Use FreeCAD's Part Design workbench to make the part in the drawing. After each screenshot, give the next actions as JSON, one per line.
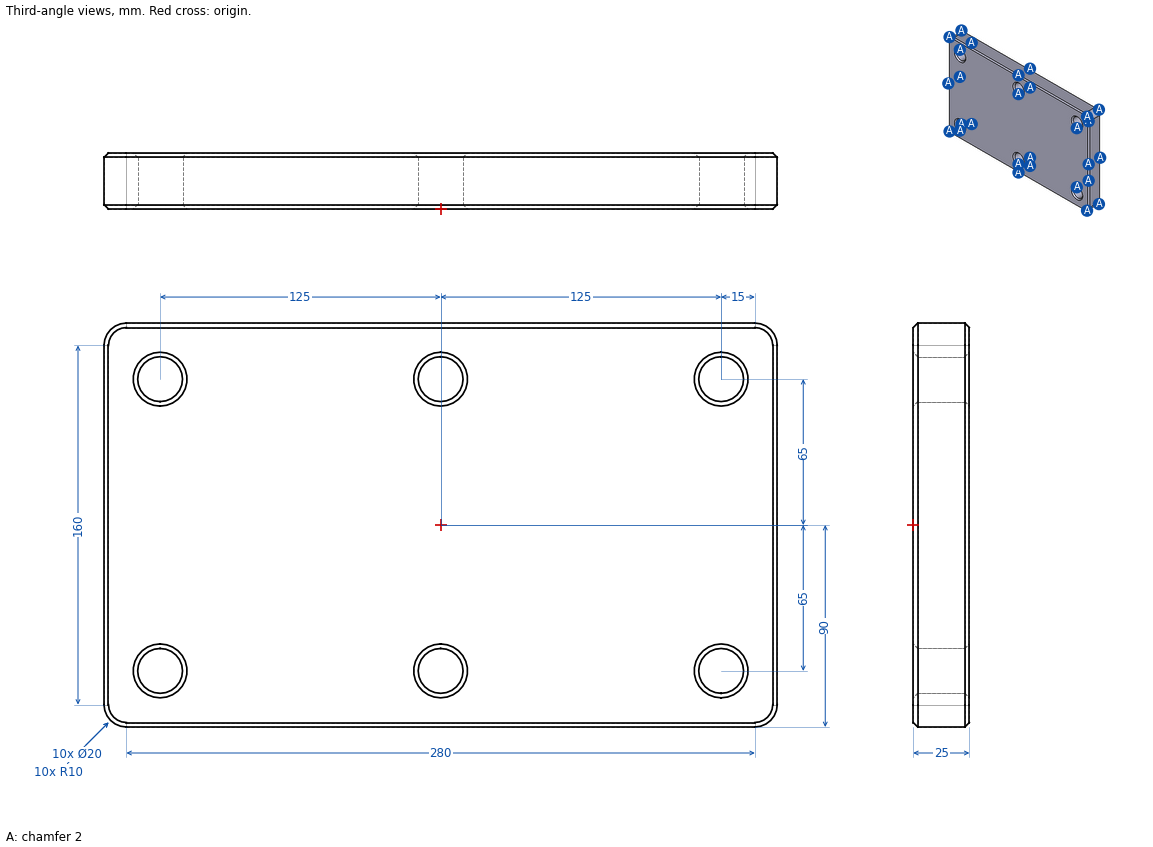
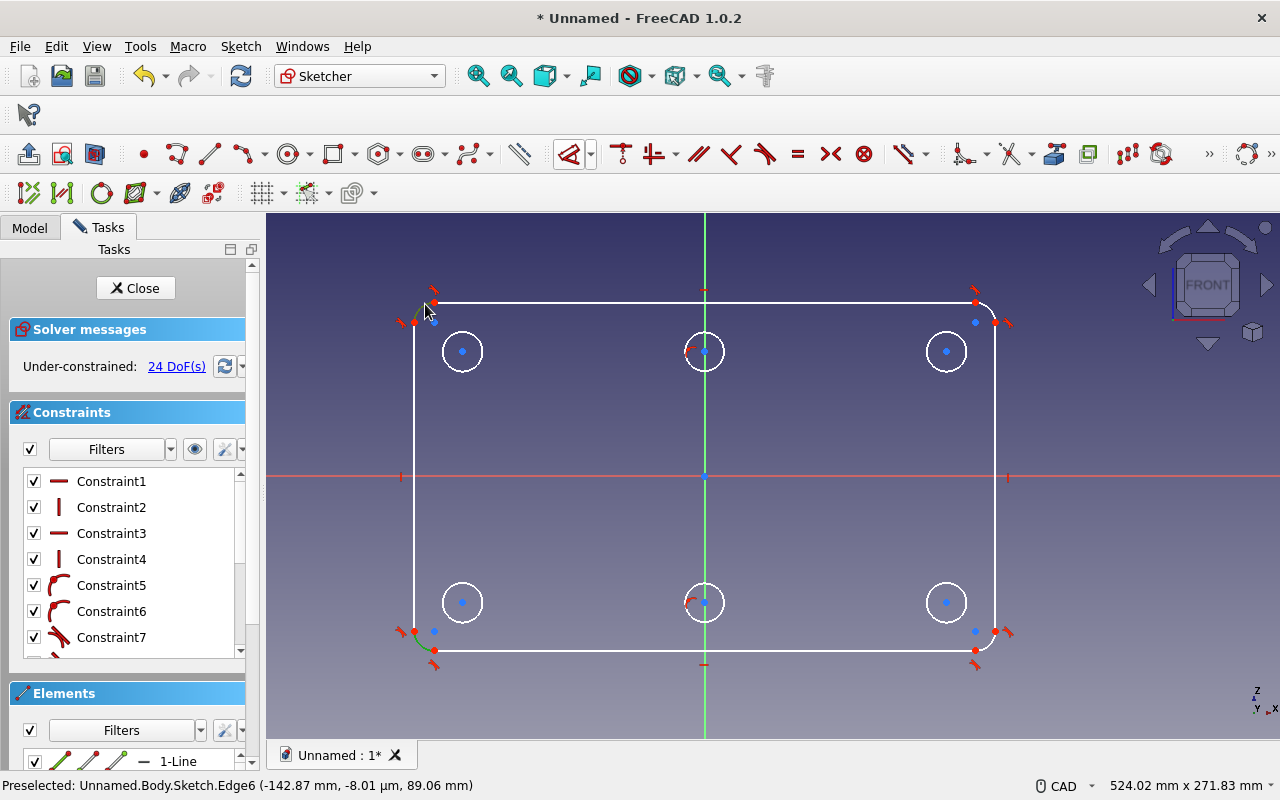
{"action": "scroll", "coordinate": [993, 314], "scroll_direction": "up", "scroll_amount": 2}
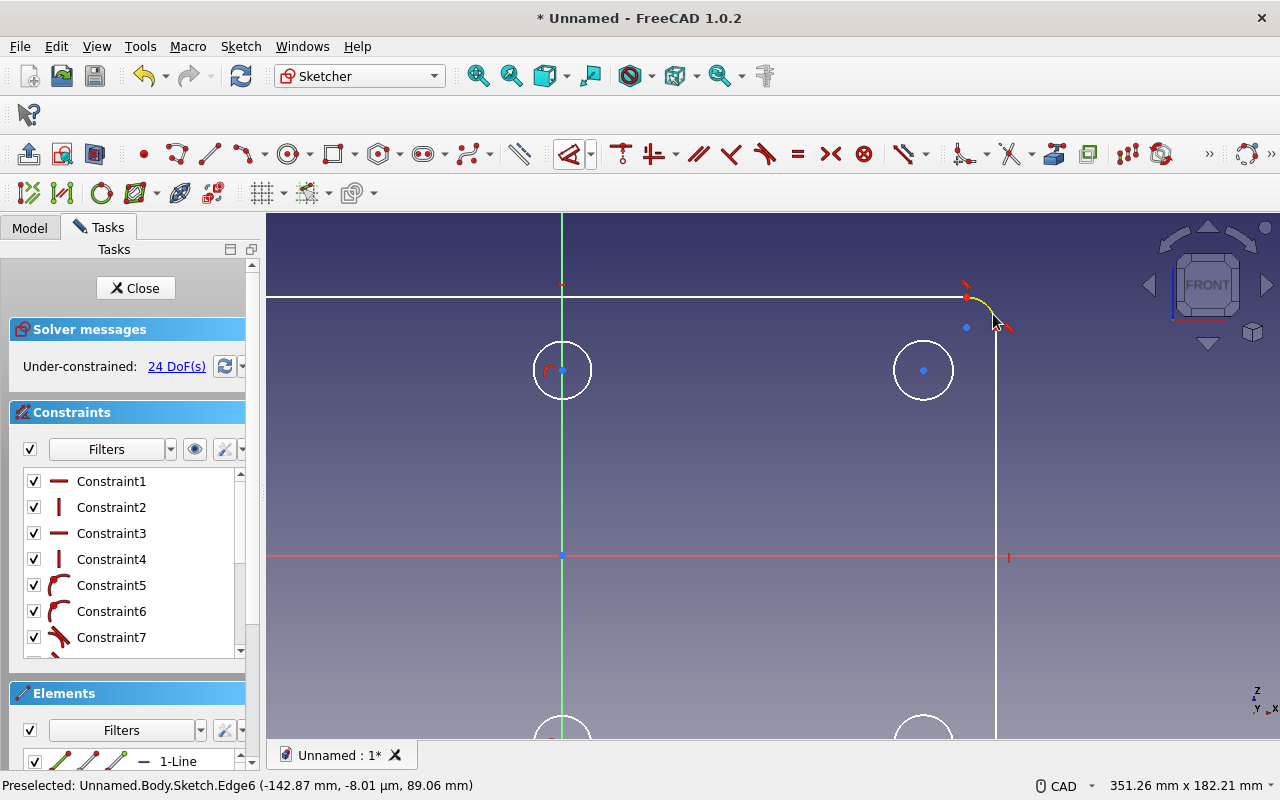
{"action": "left_click", "coordinate": [993, 313]}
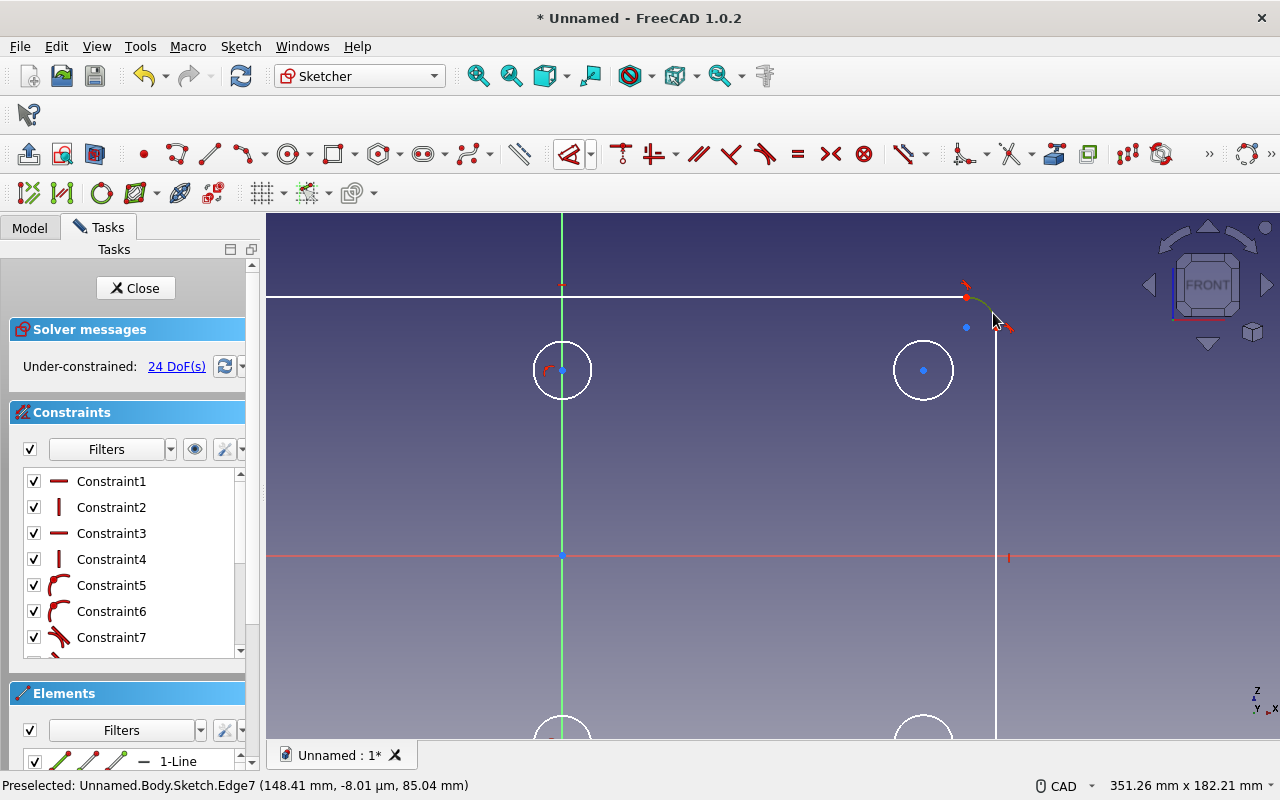
{"action": "scroll", "coordinate": [993, 314], "scroll_direction": "down", "scroll_amount": 2}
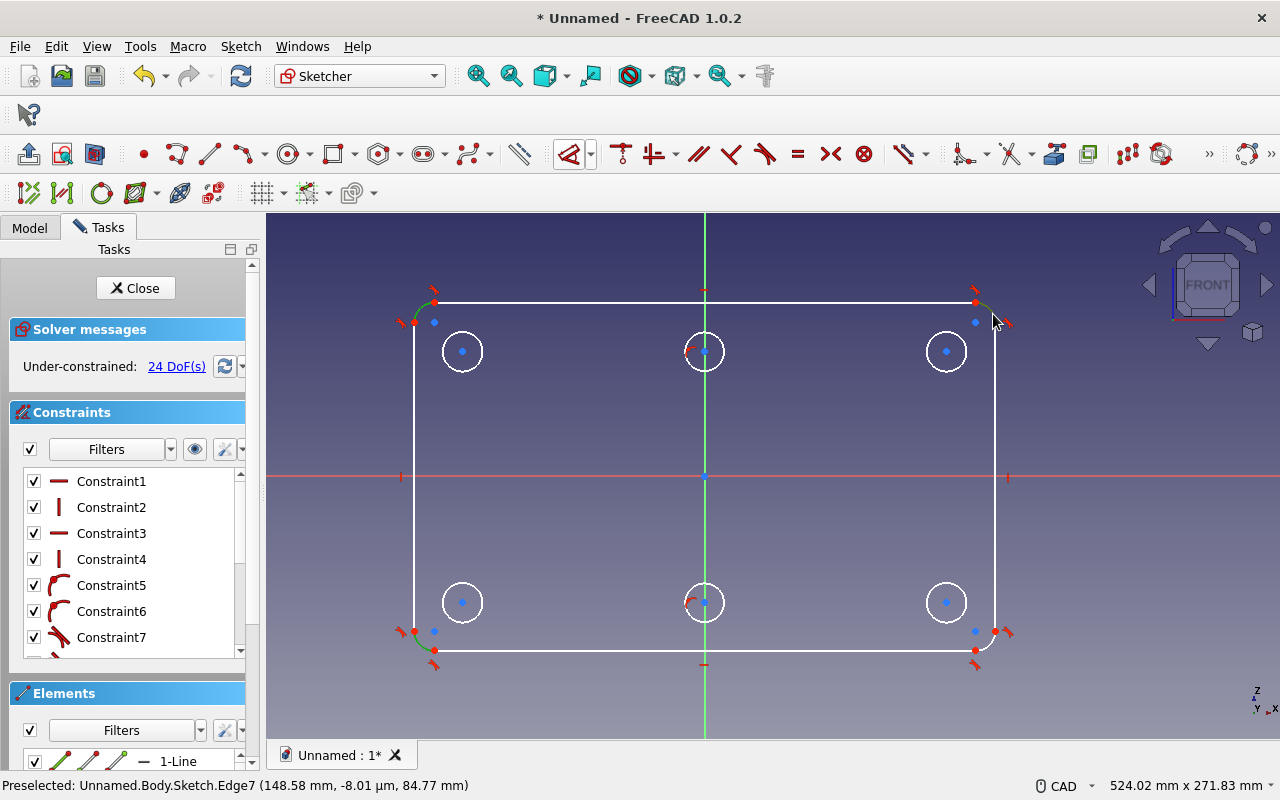
{"action": "scroll", "coordinate": [985, 649], "scroll_direction": "up", "scroll_amount": 3}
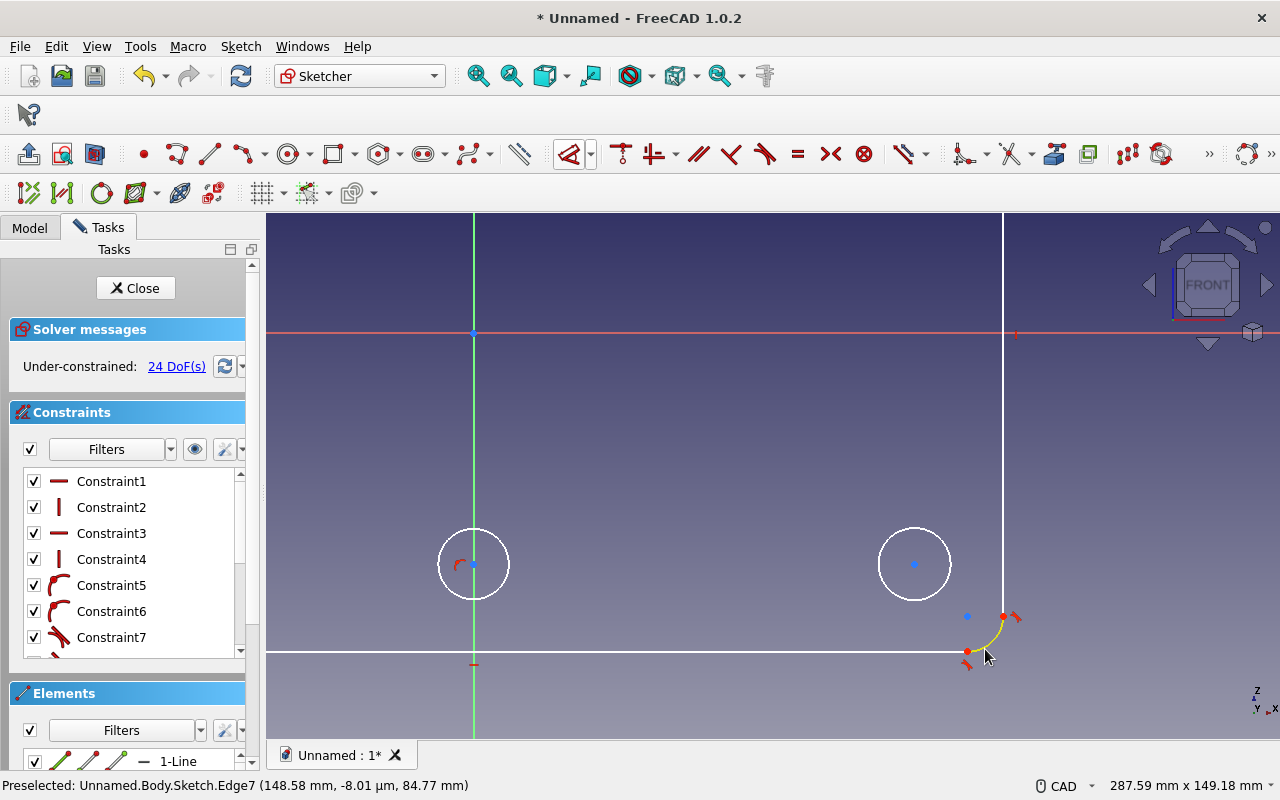
{"action": "left_click", "coordinate": [984, 648]}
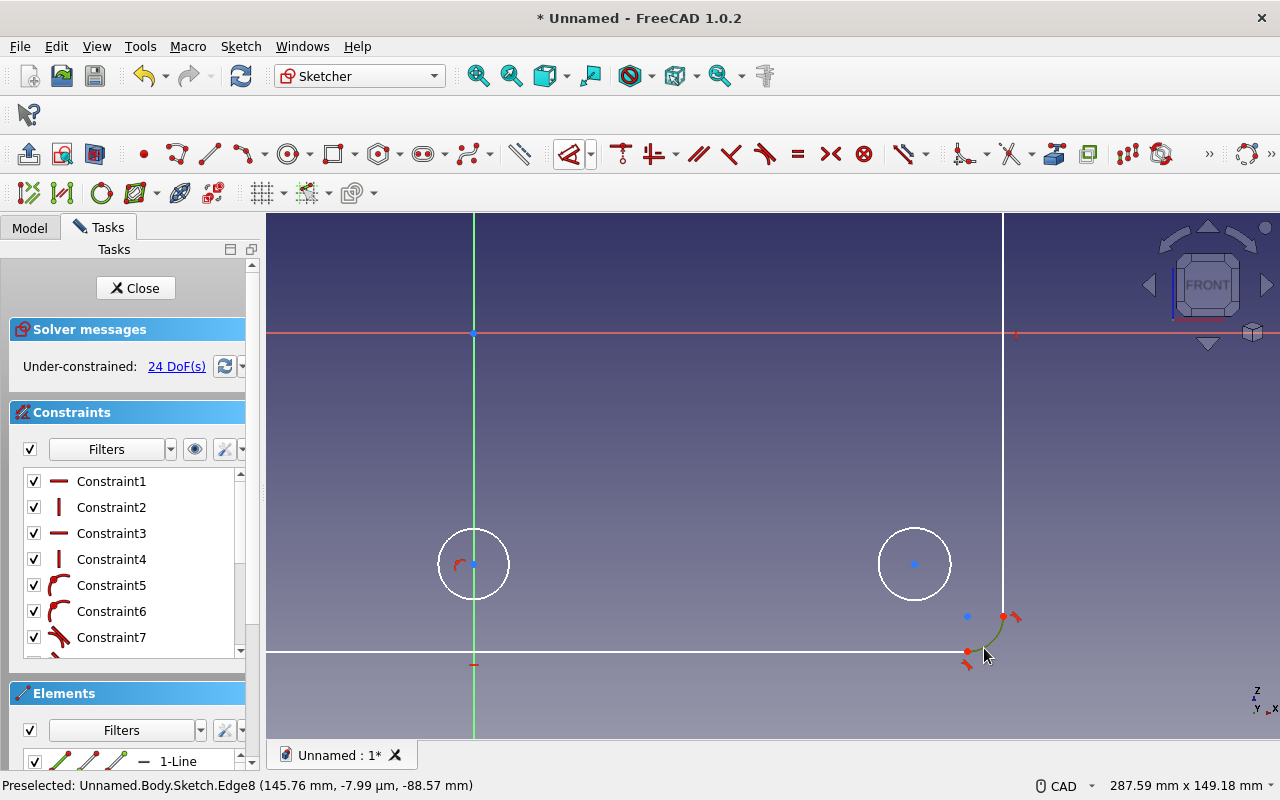
{"action": "left_click", "coordinate": [798, 154]}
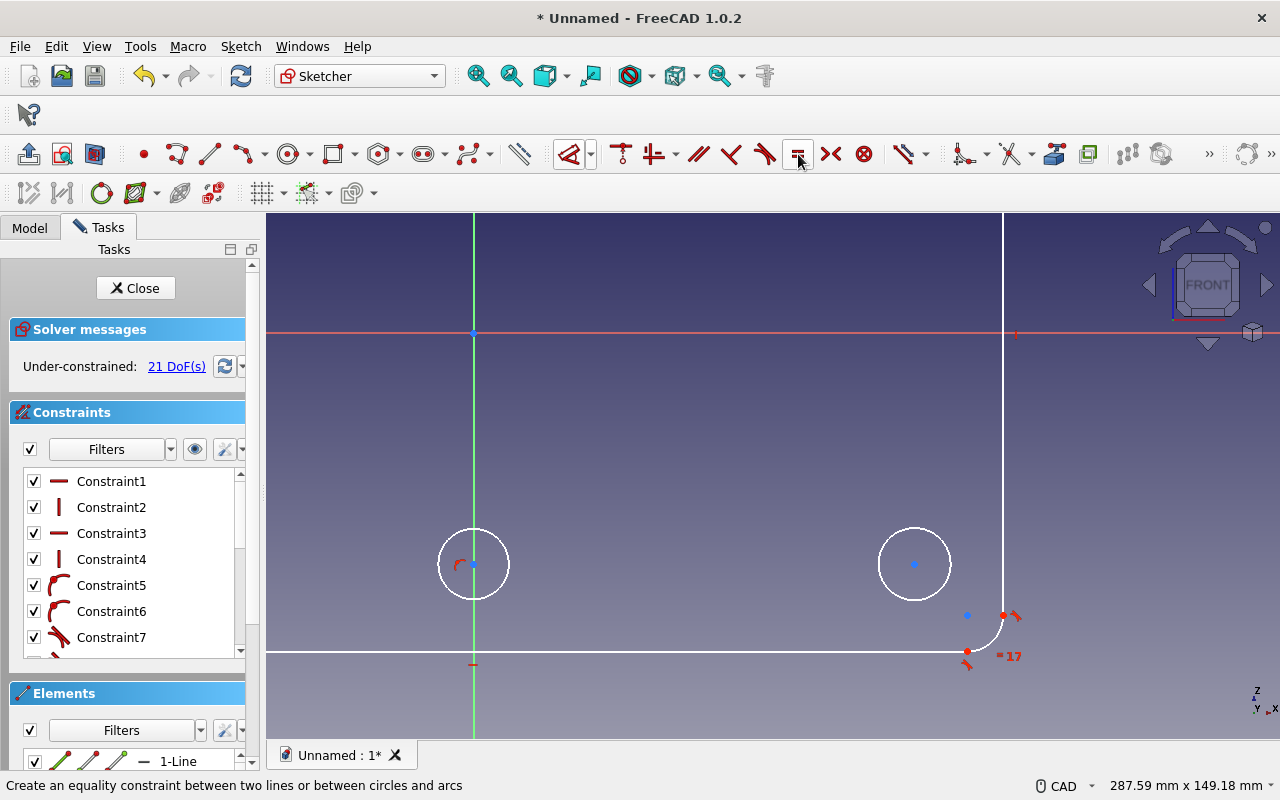
{"action": "scroll", "coordinate": [985, 650], "scroll_direction": "down", "scroll_amount": 3}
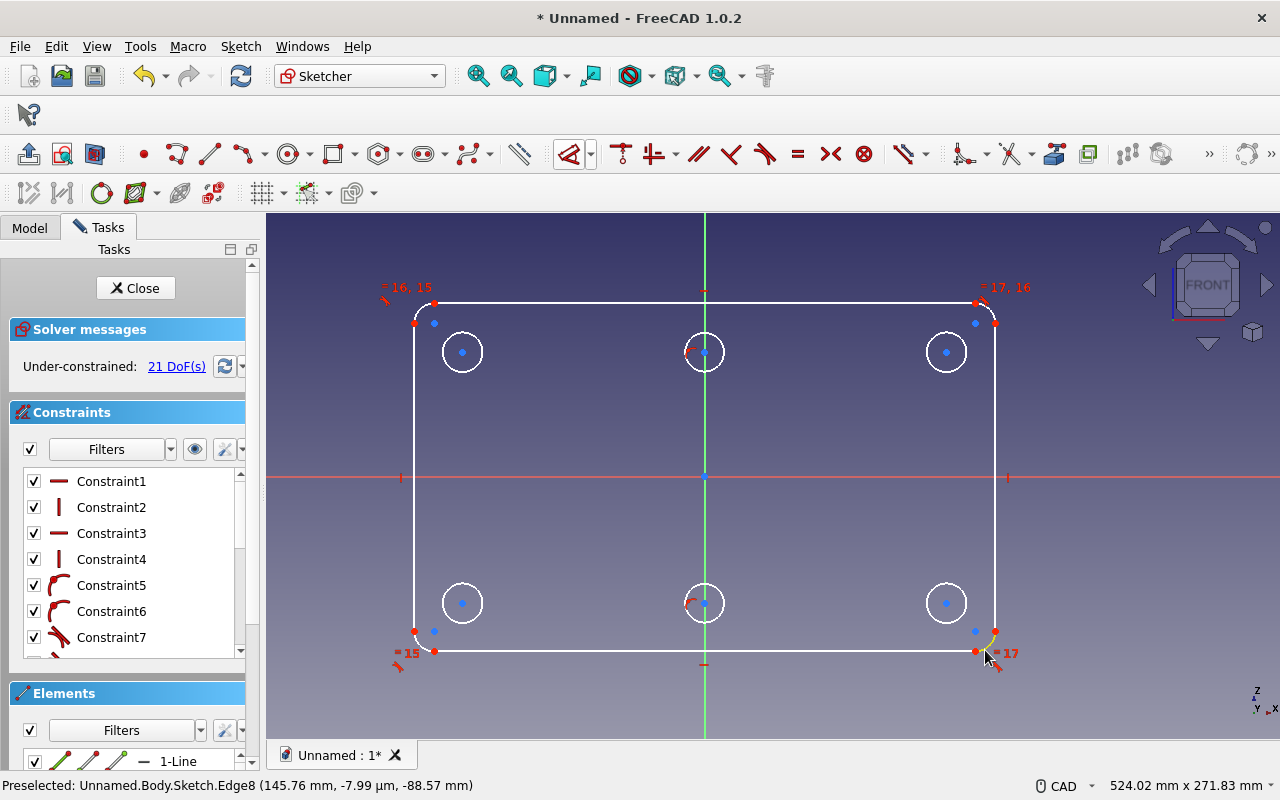
{"action": "left_click", "coordinate": [961, 338]}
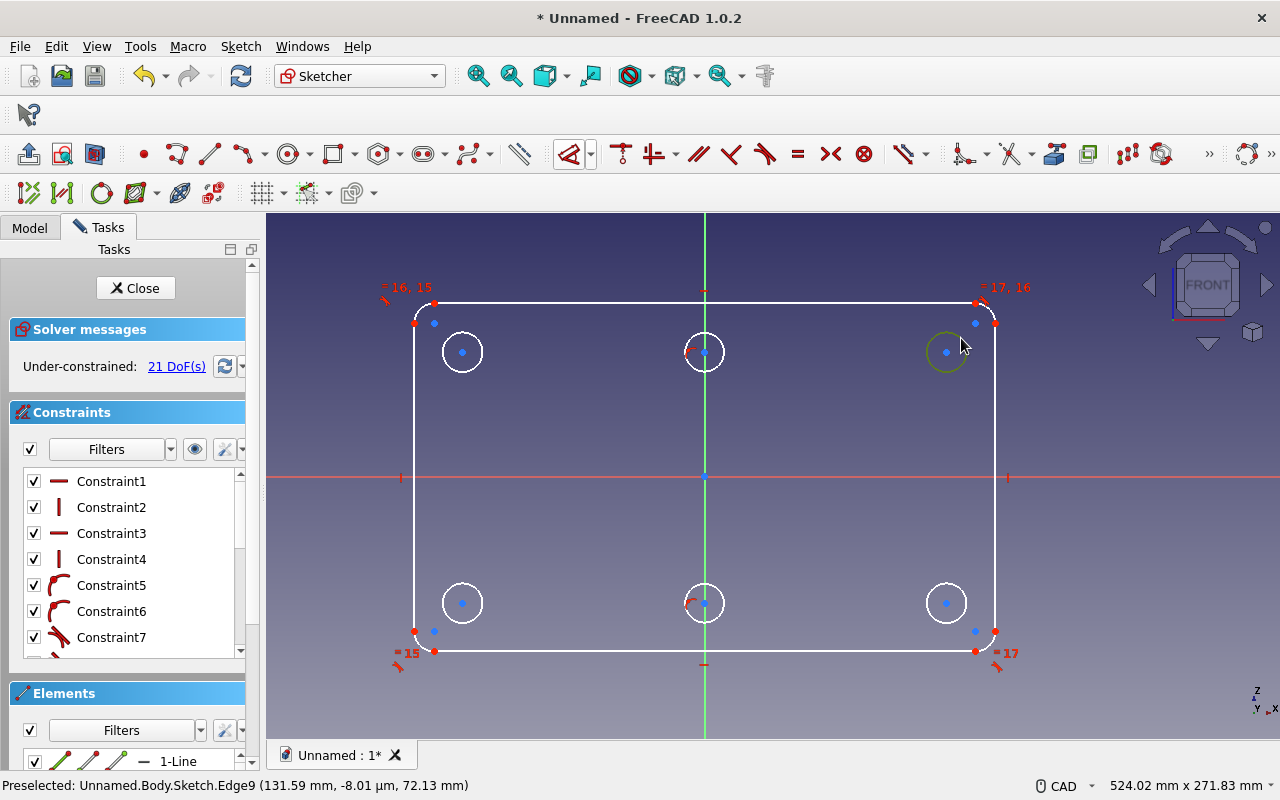
{"action": "left_click", "coordinate": [718, 339]}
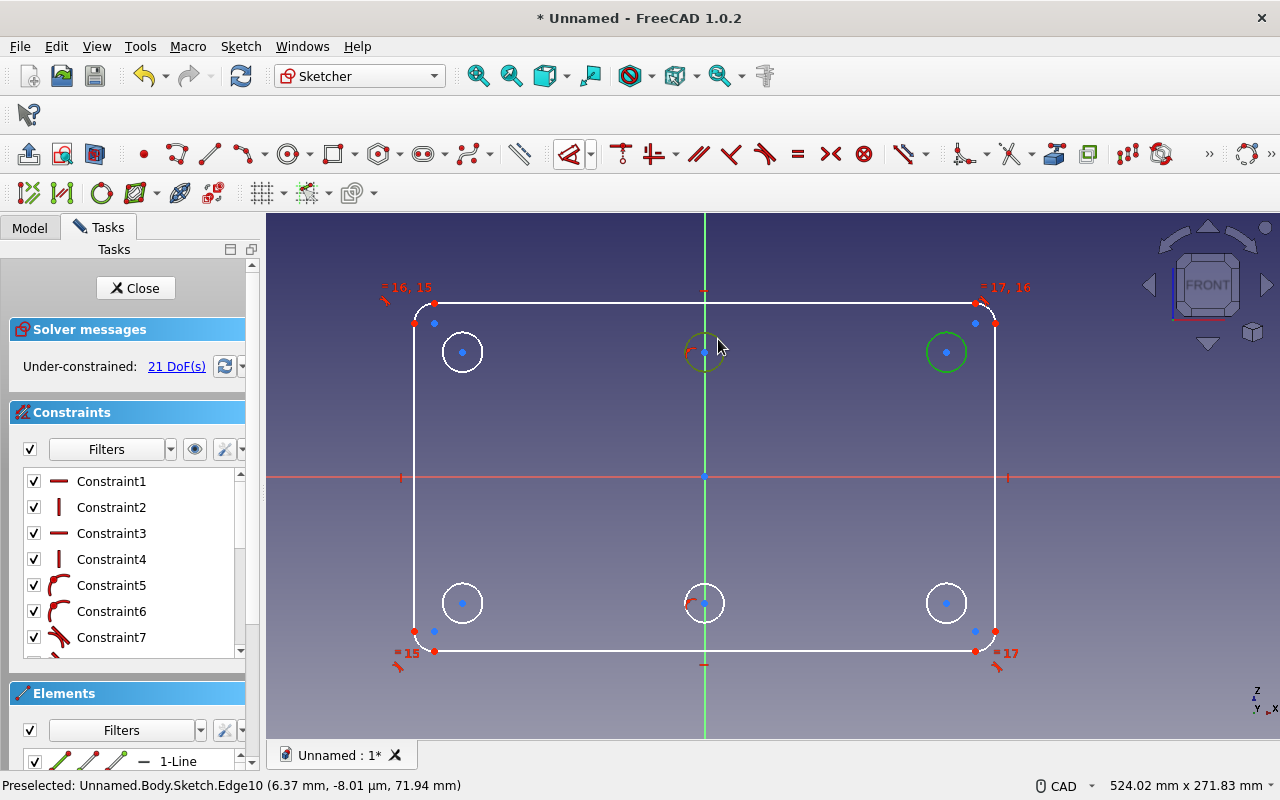
{"action": "left_click", "coordinate": [477, 338]}